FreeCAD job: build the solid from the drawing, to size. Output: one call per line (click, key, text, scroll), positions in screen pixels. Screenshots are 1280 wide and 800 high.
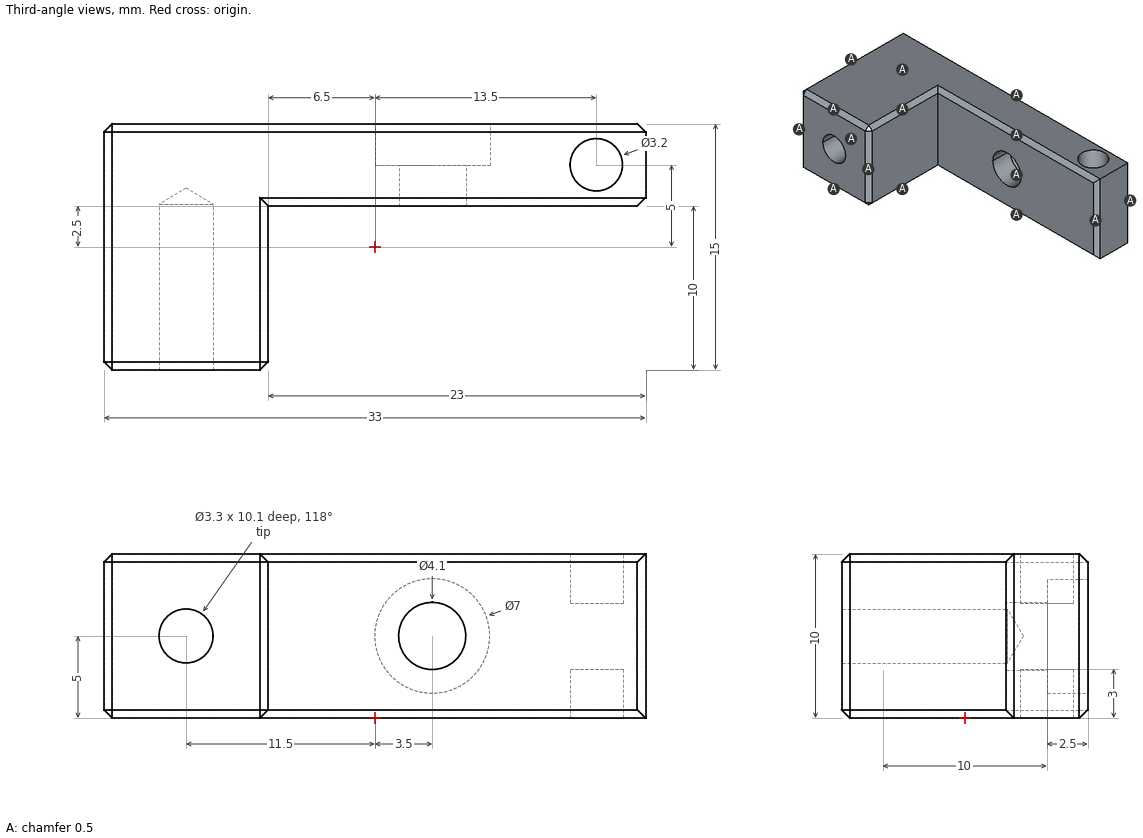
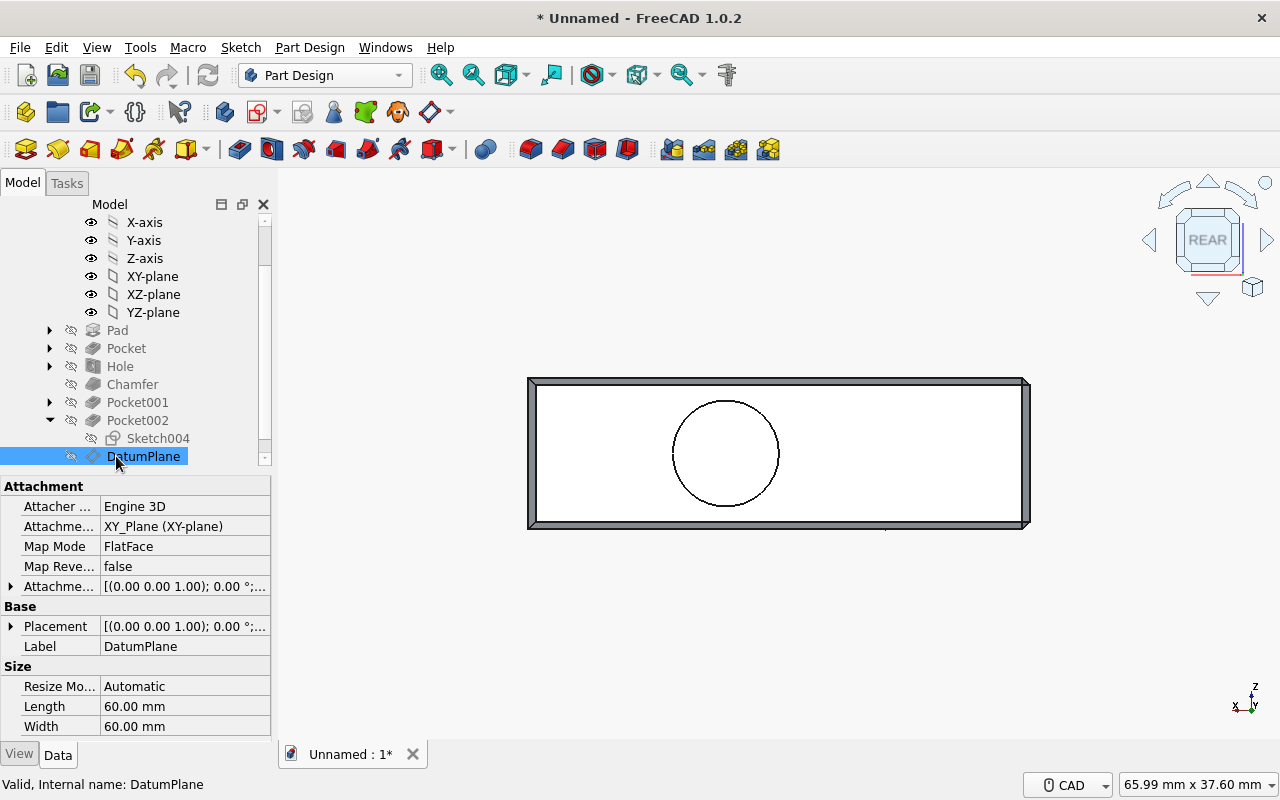
click(726, 452)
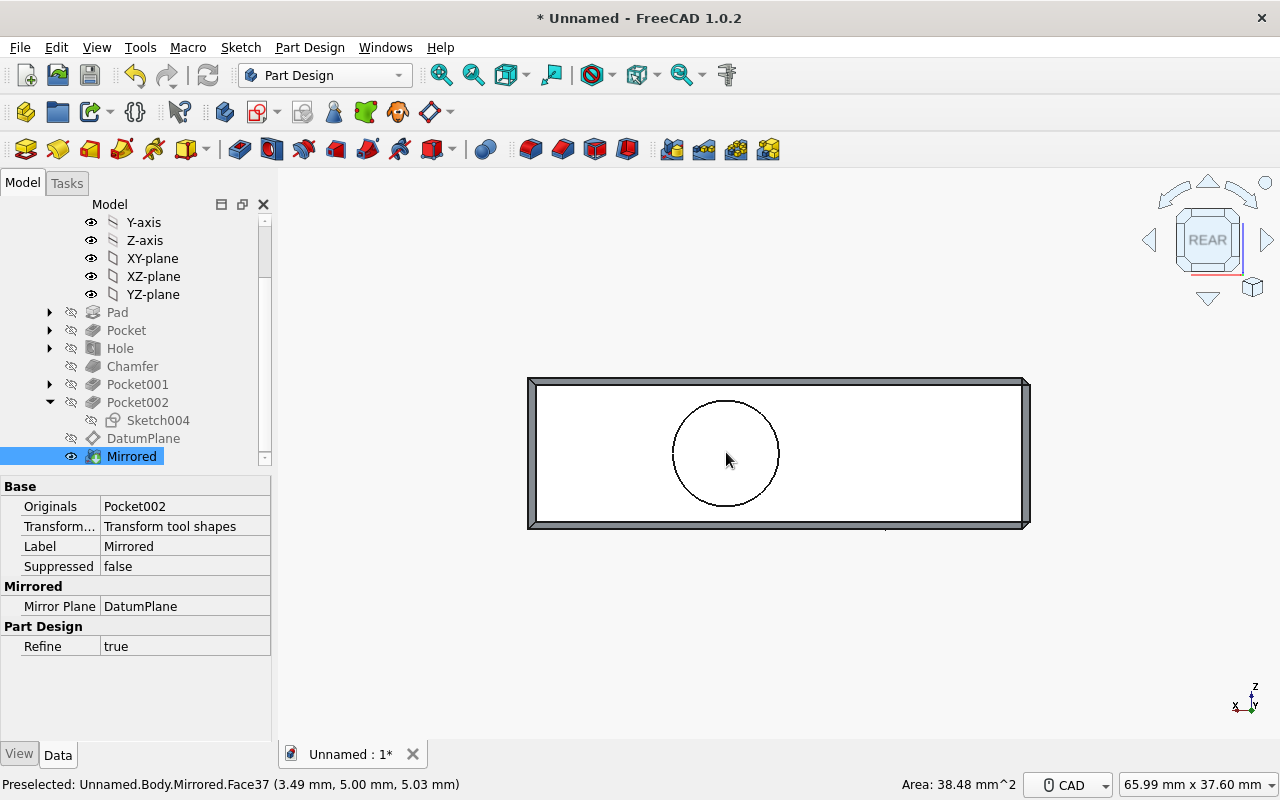
click(258, 112)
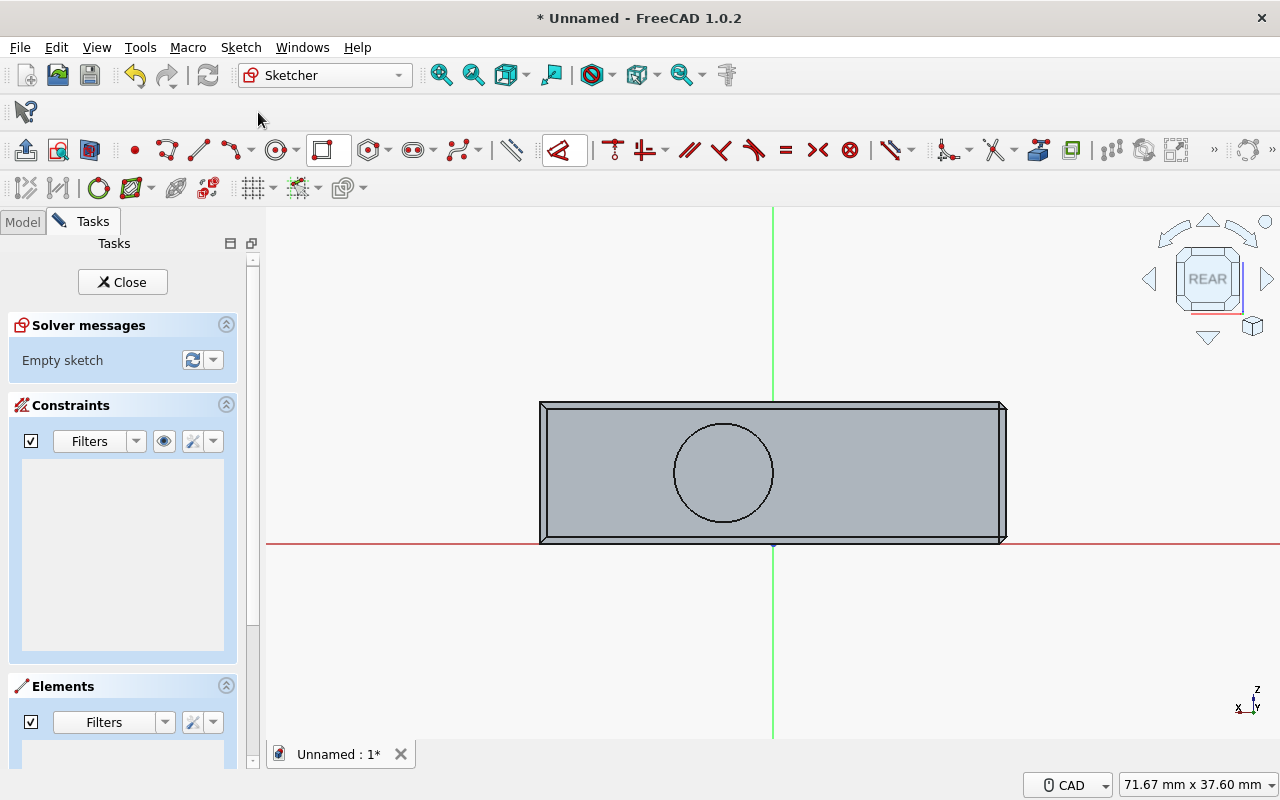
scroll(746, 503, up, 6)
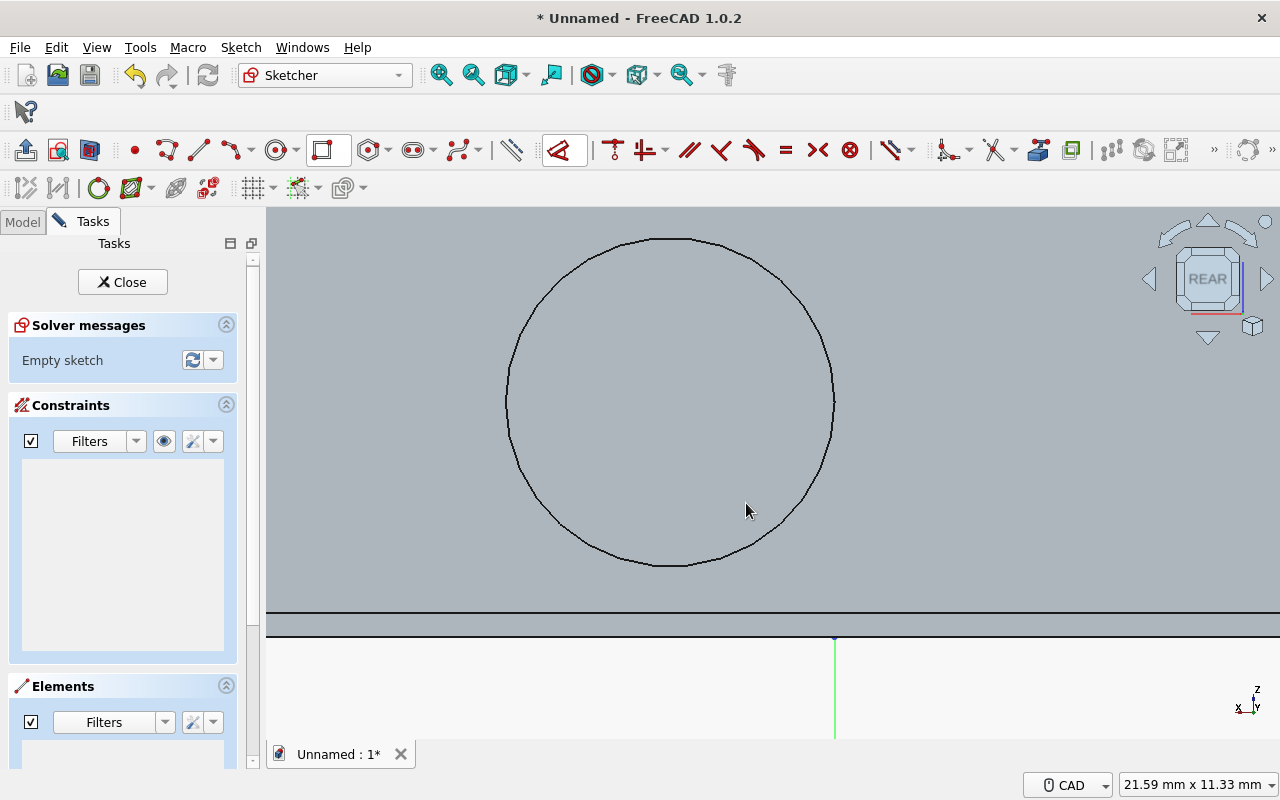
click(276, 150)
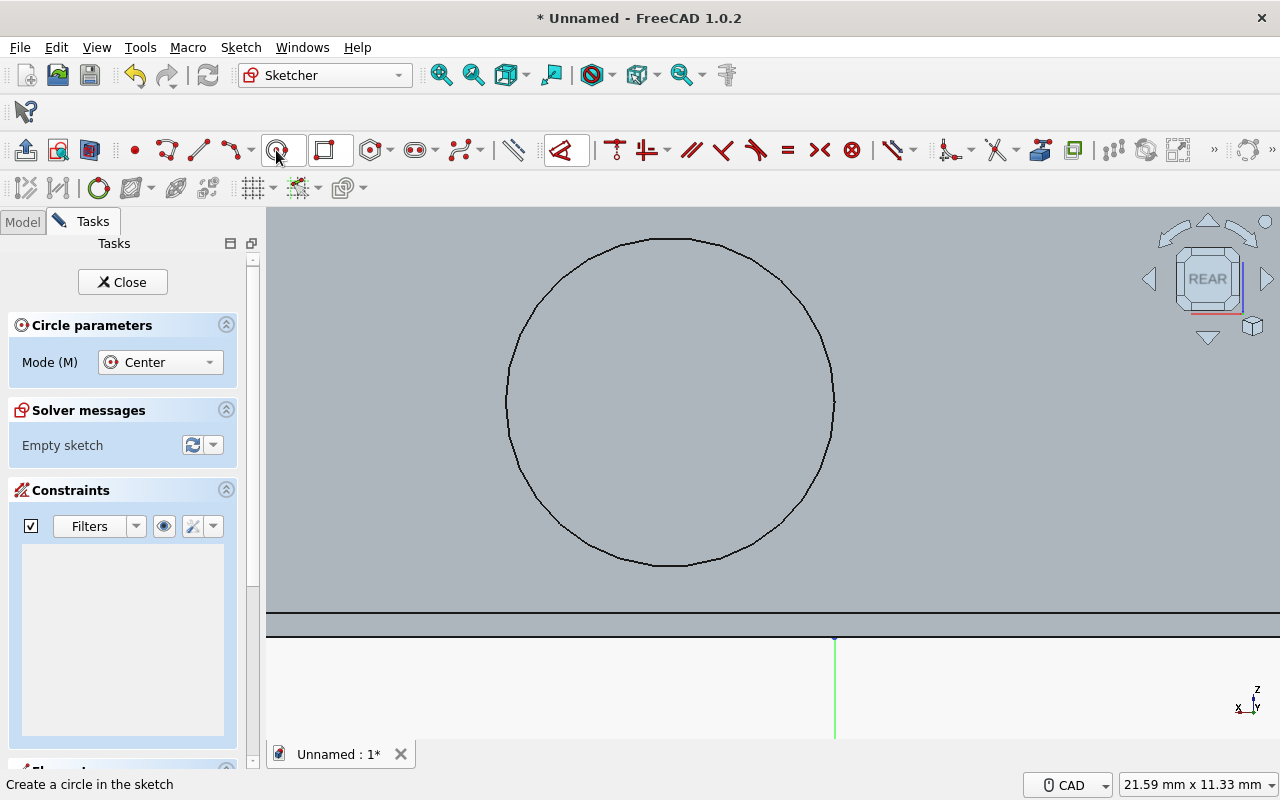
click(670, 402)
move(738, 334)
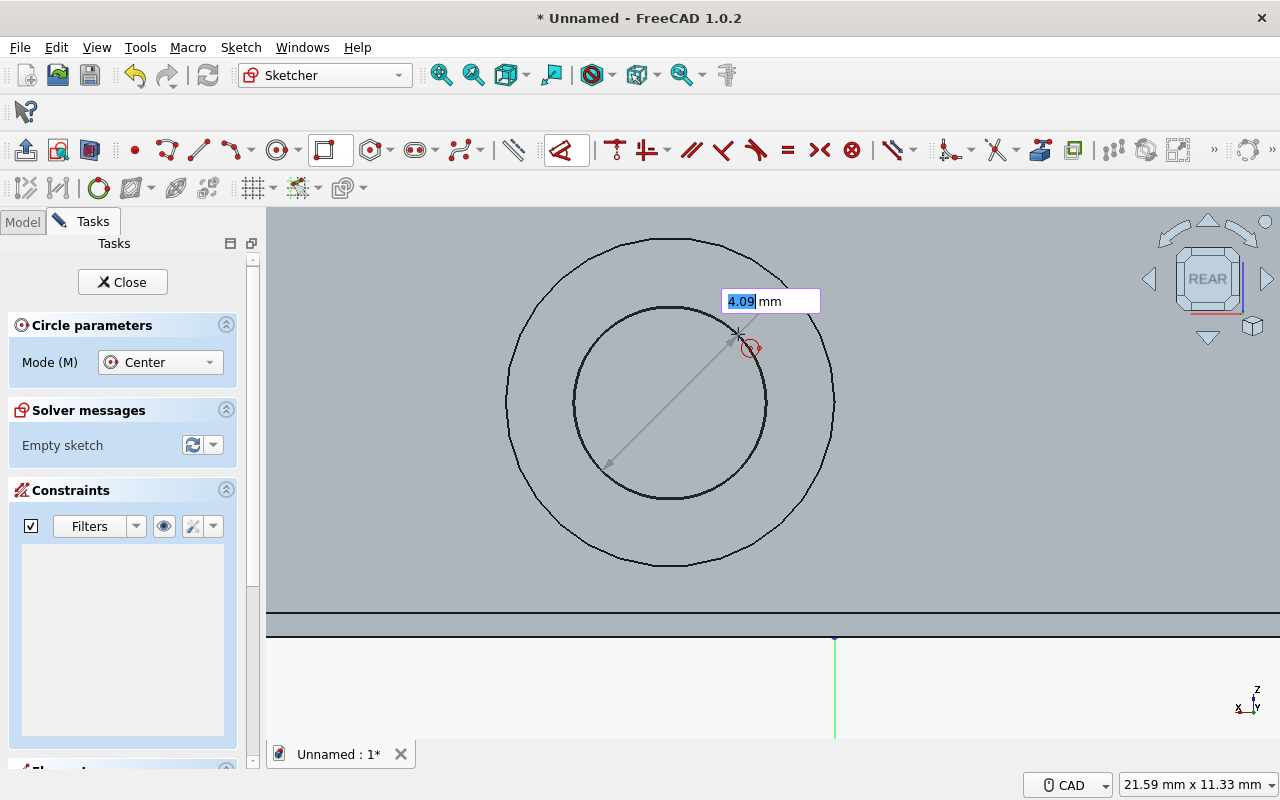
text(4.1)
key(Return)
key(Escape)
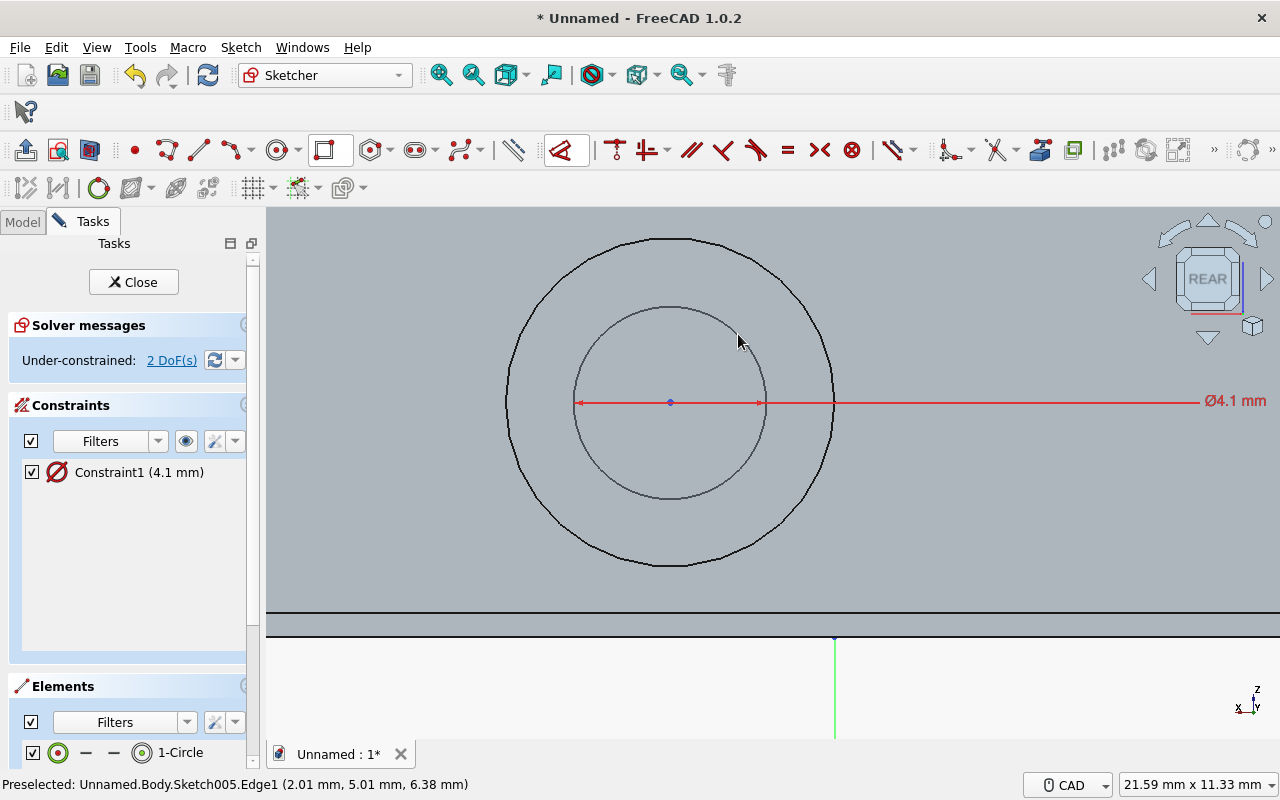
click(670, 403)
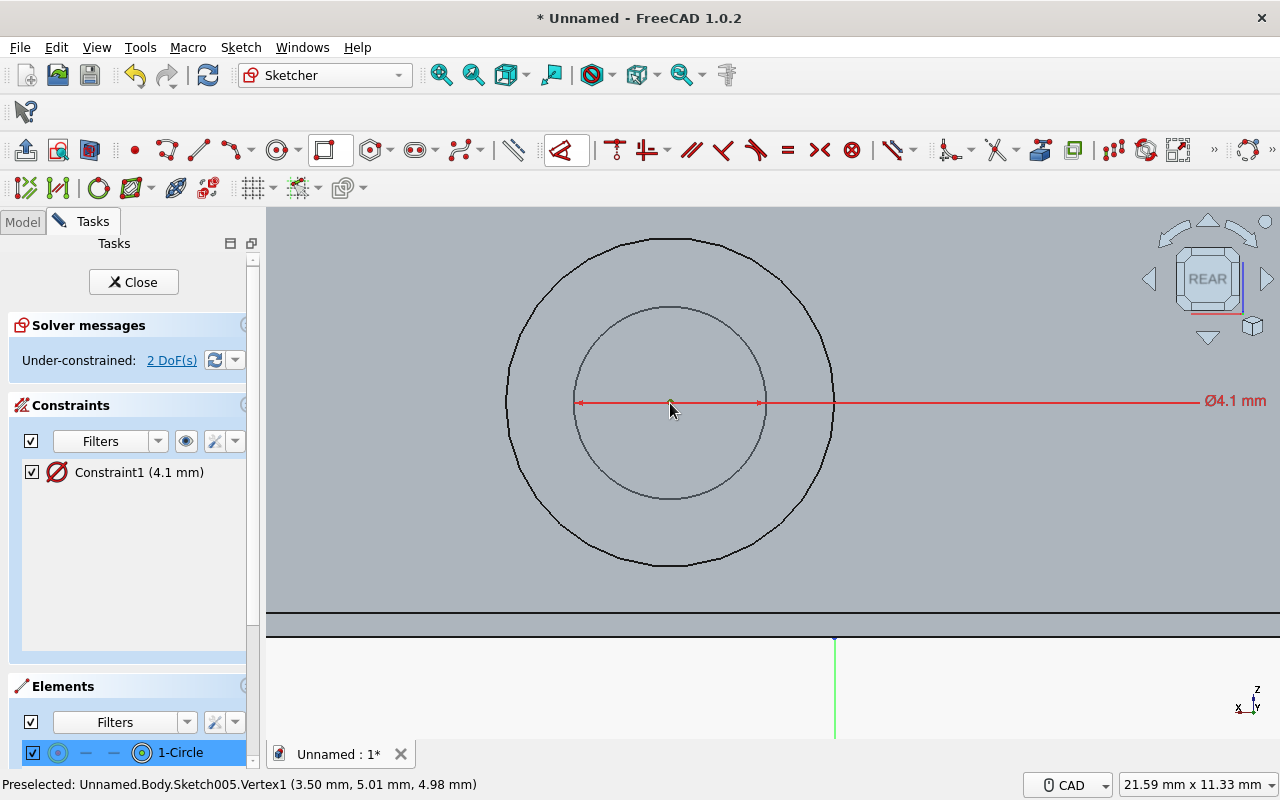
click(584, 150)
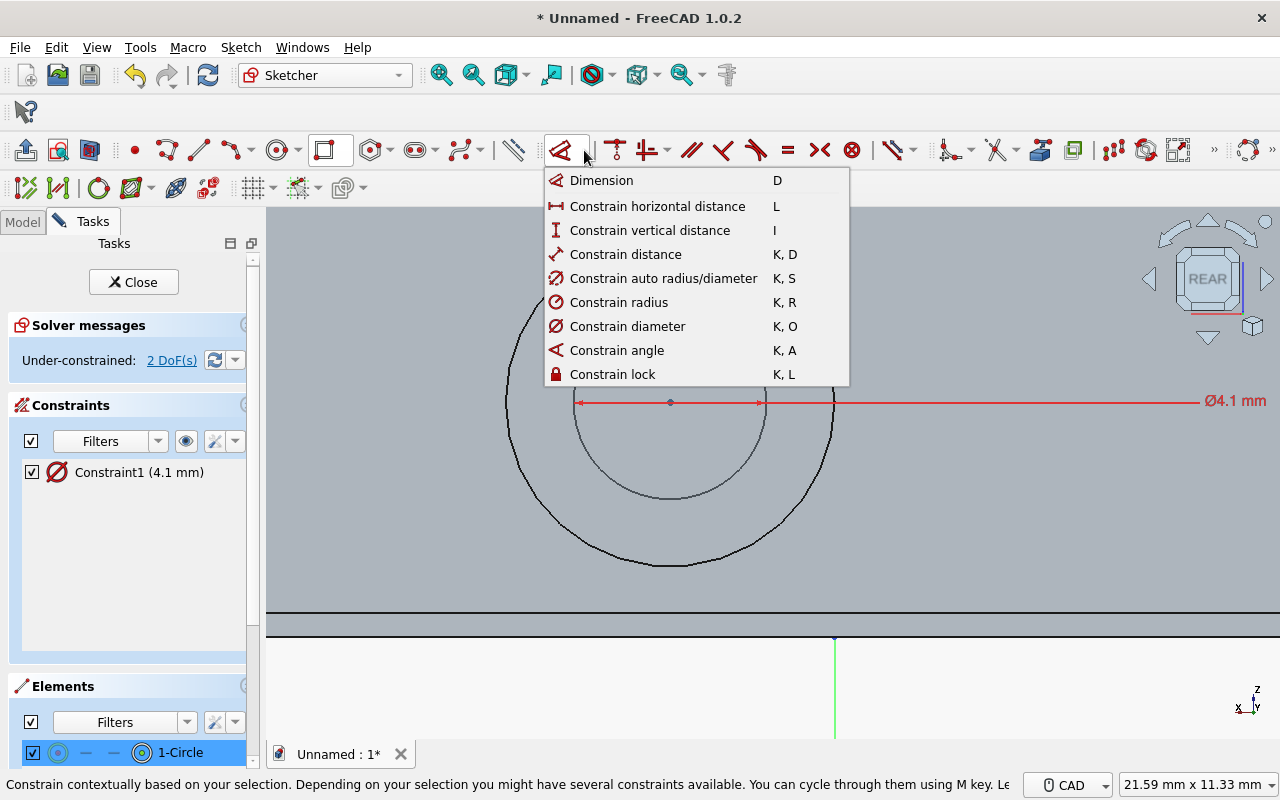
click(697, 230)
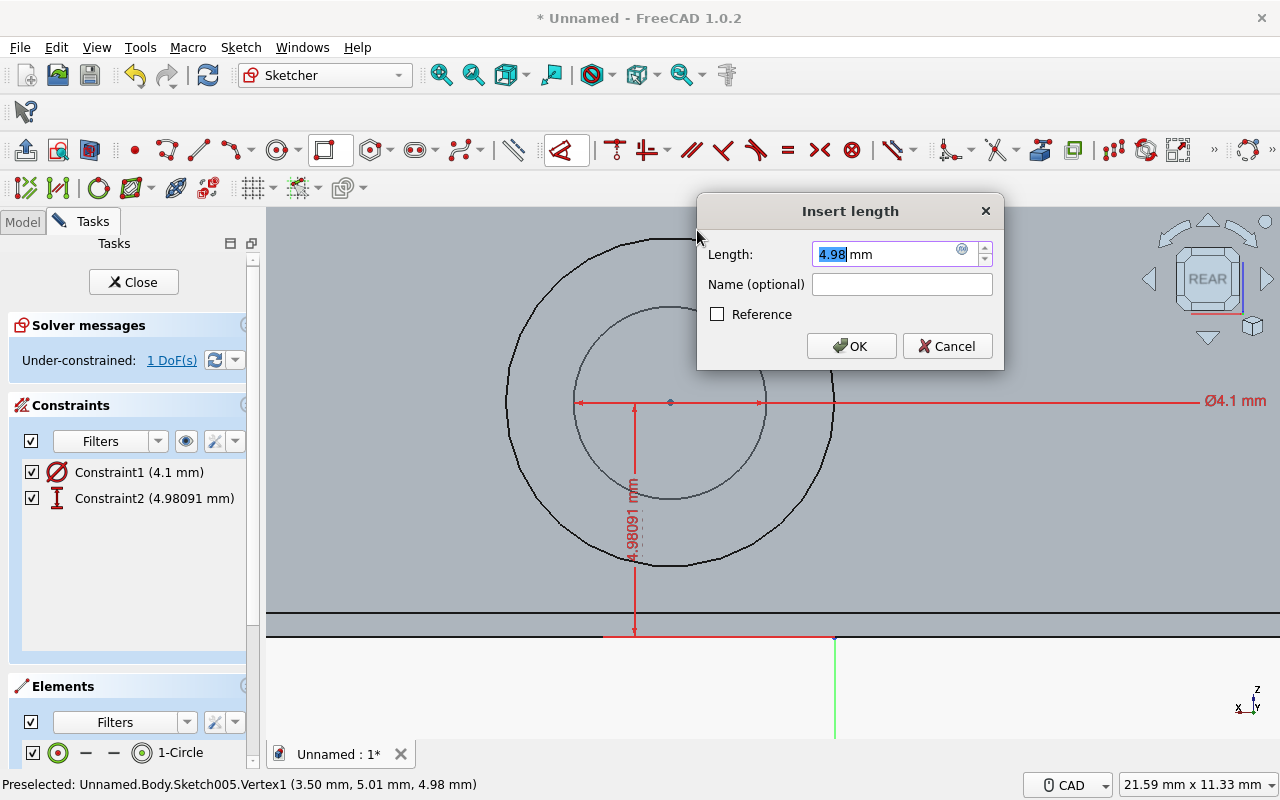
text(5)
key(Return)